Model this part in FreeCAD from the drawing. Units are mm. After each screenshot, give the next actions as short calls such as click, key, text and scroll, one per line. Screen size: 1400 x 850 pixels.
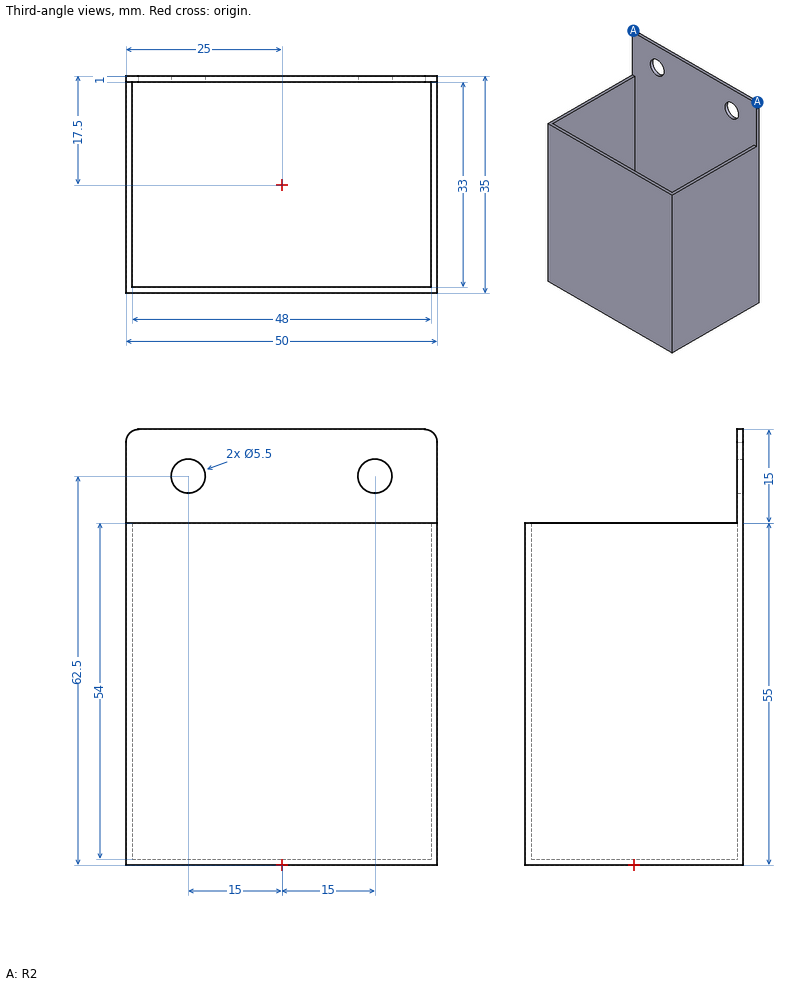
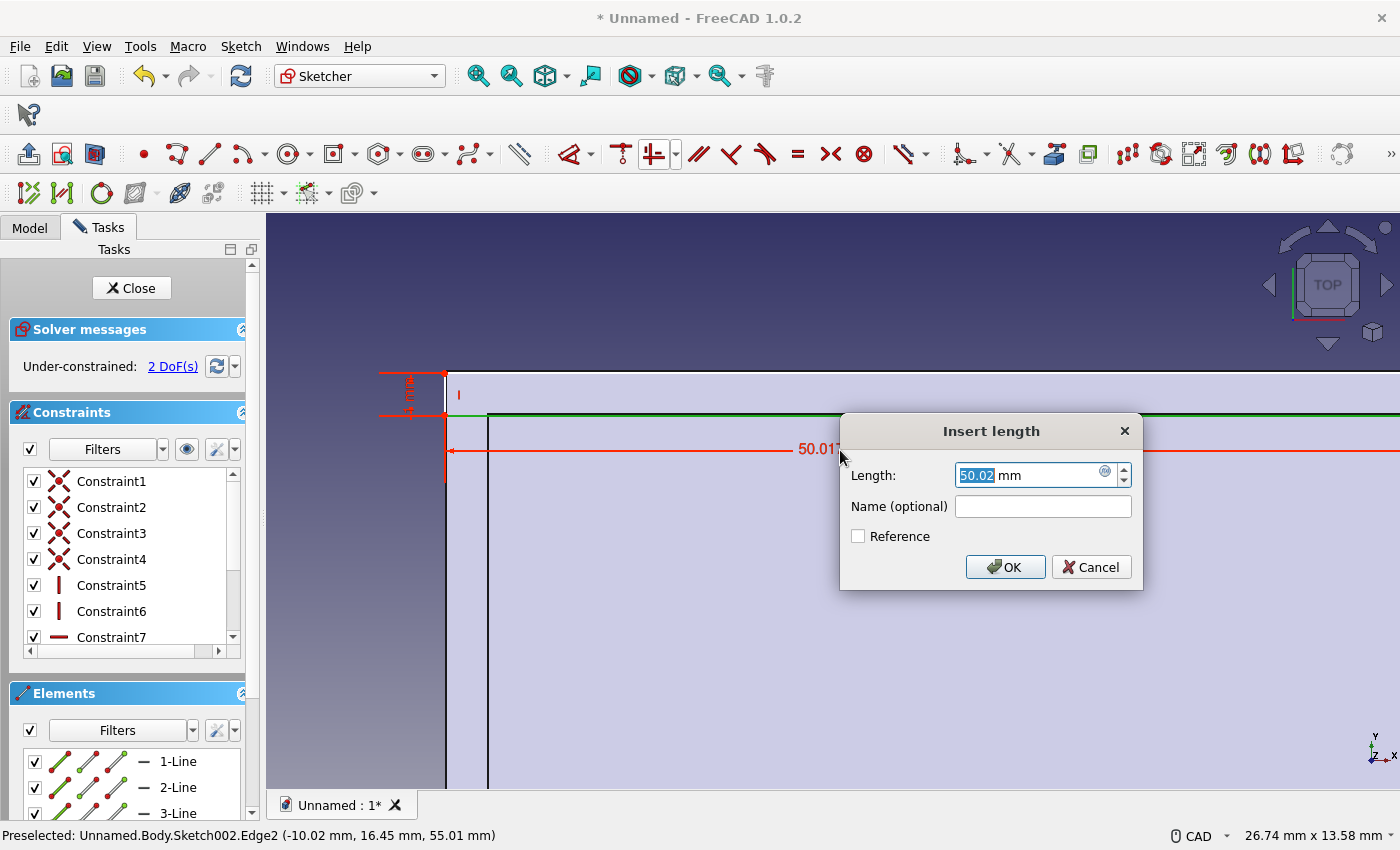
text(50)
key(Return)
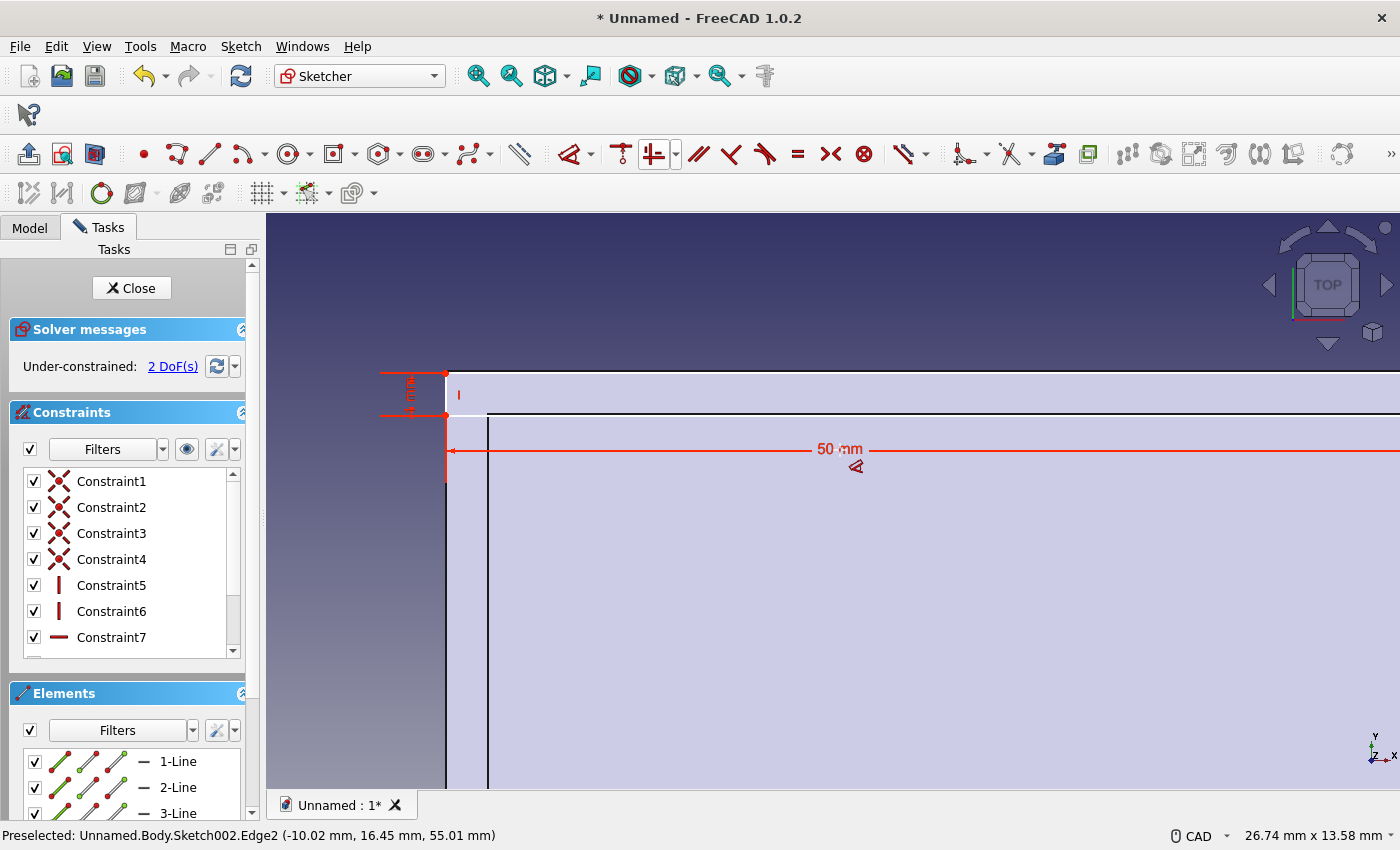
click(446, 373)
click(840, 339)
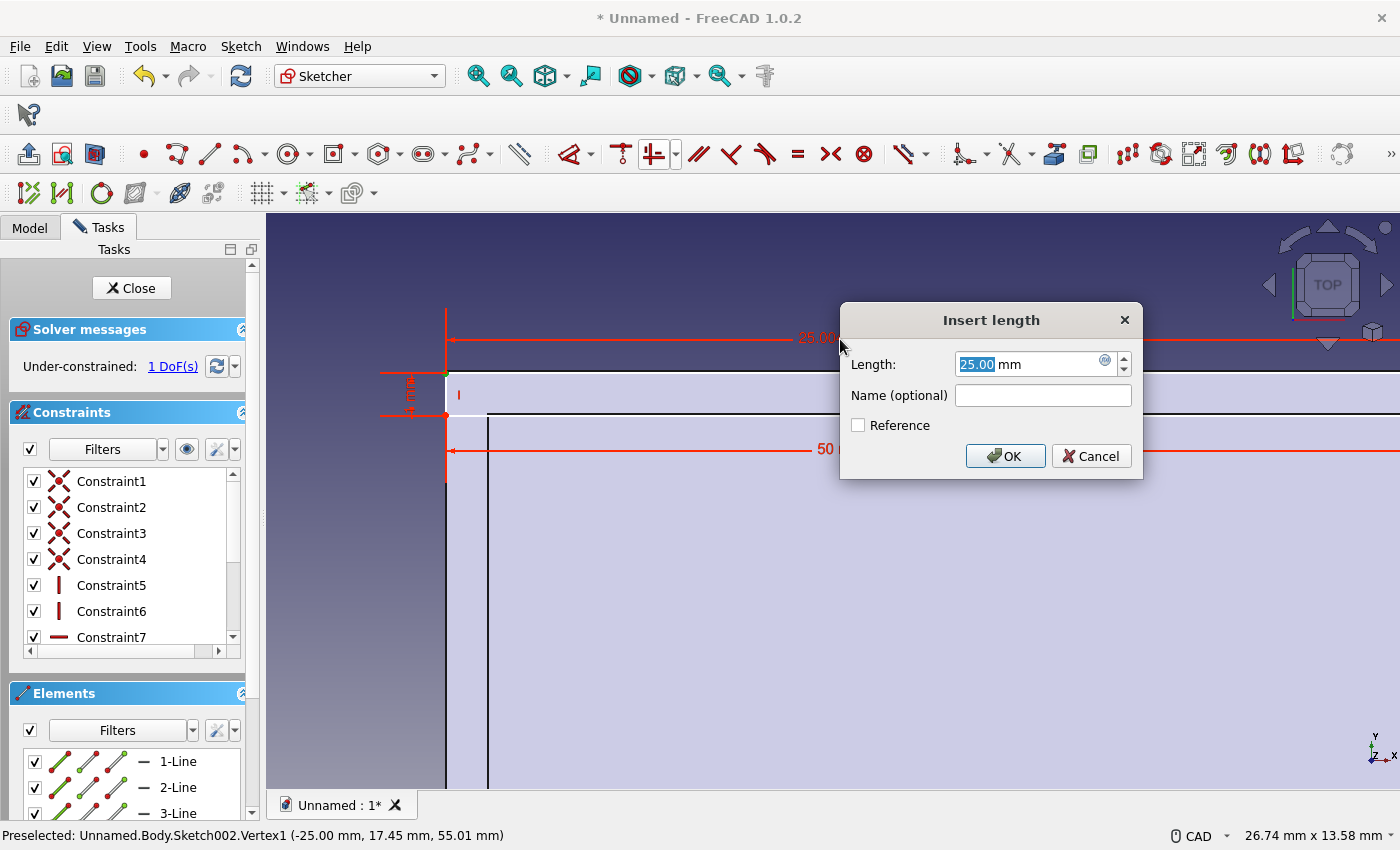
text(25)
key(Return)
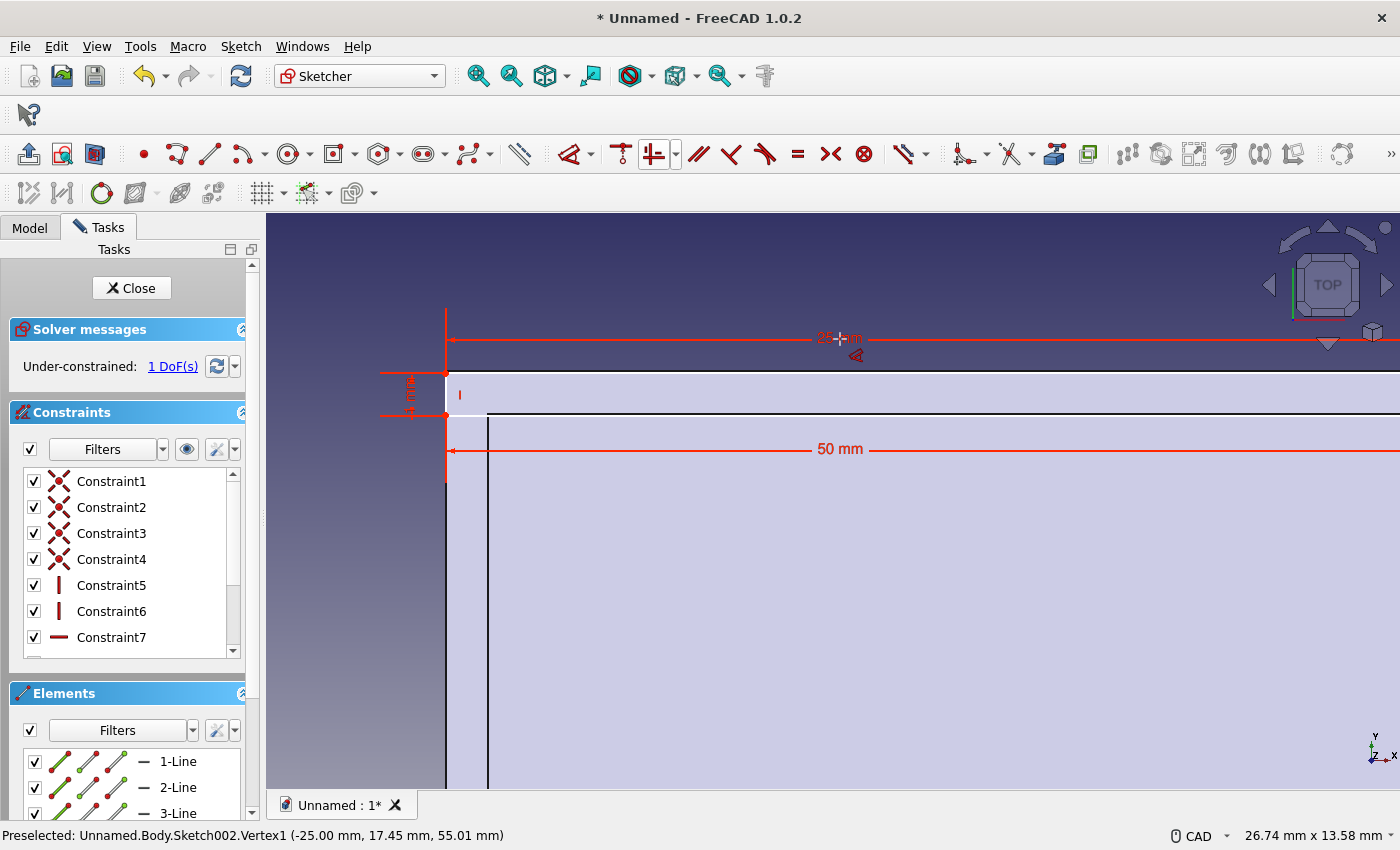
click(446, 373)
click(412, 567)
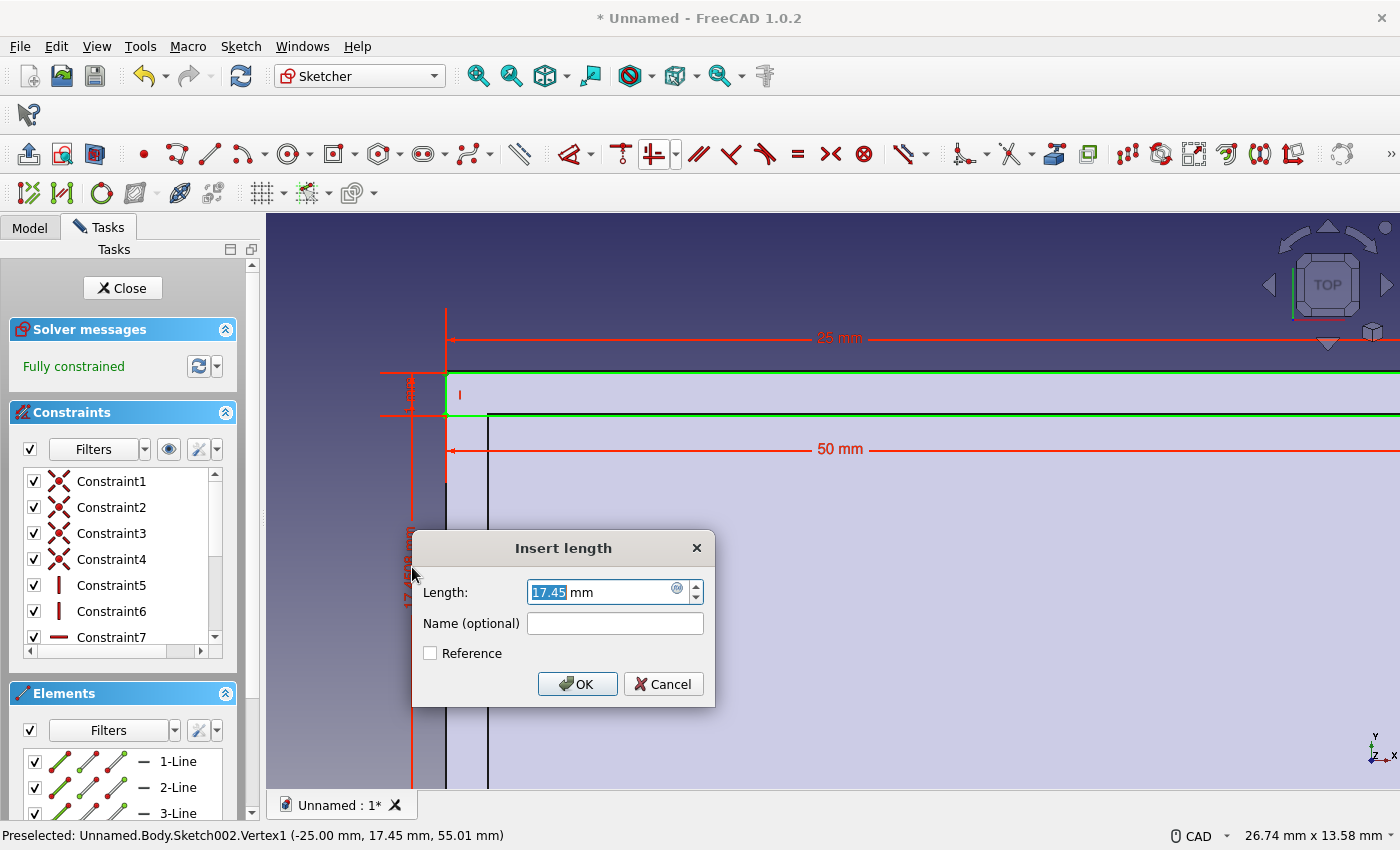
text(17.5)
key(Return)
key(Escape)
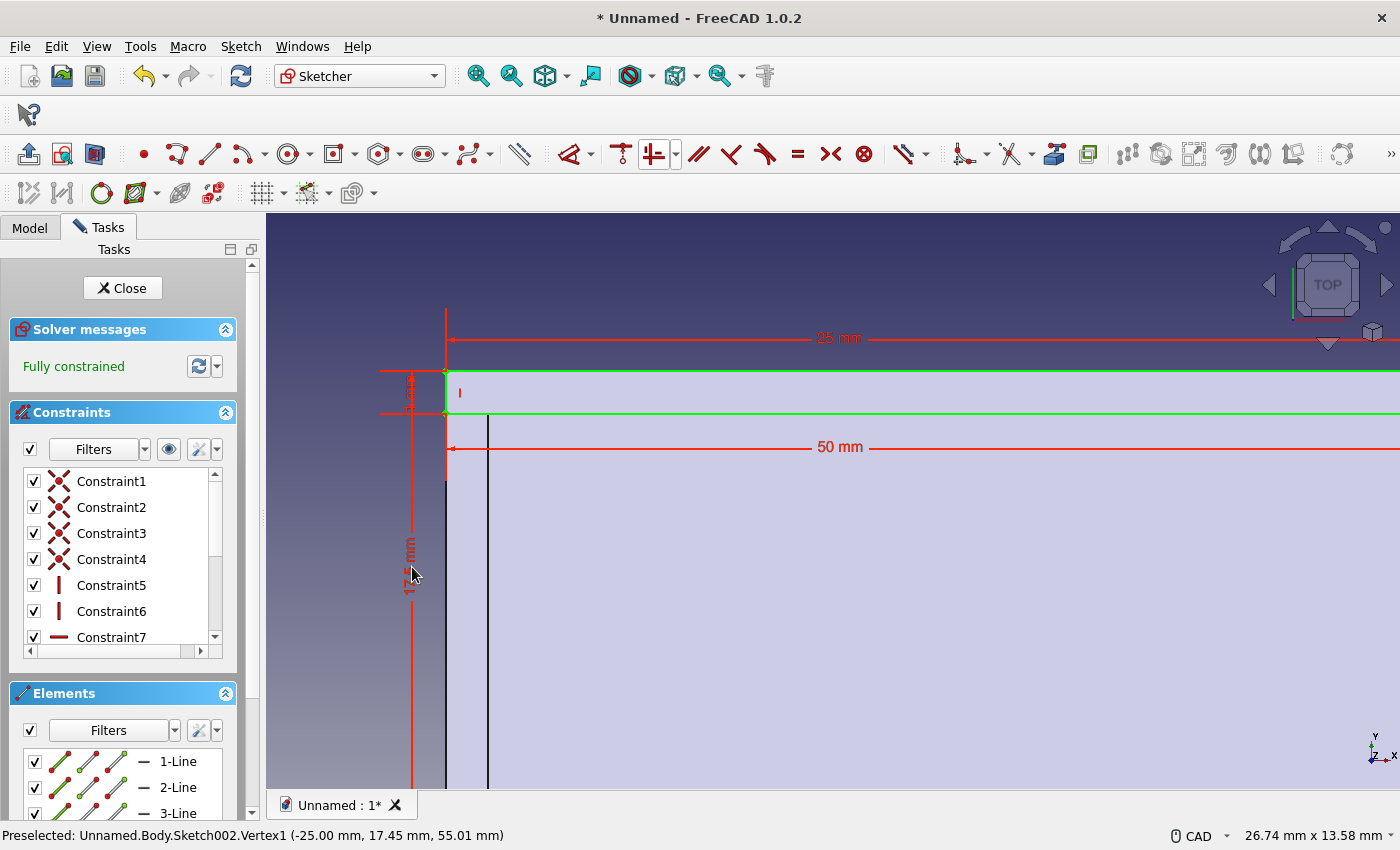
click(123, 288)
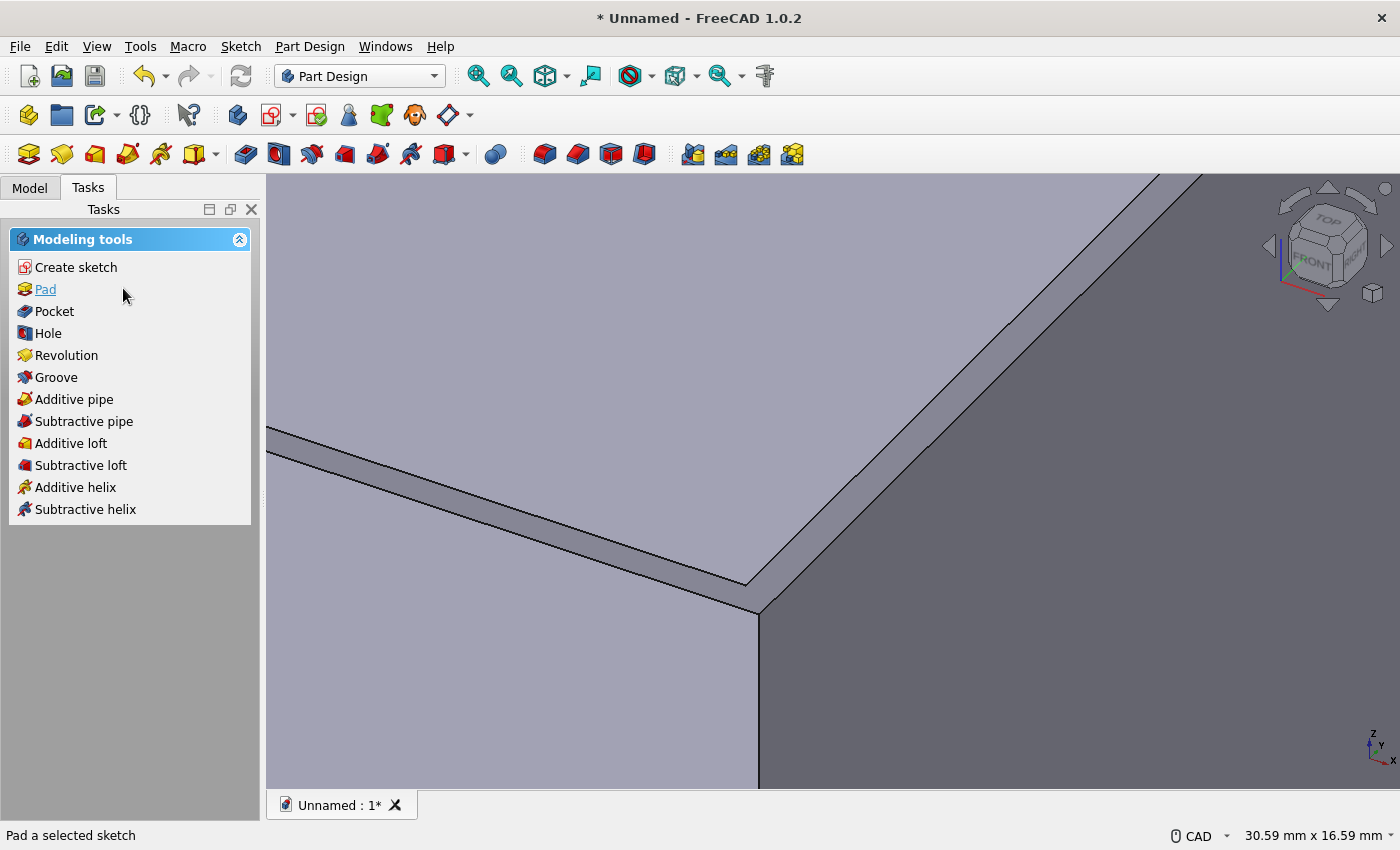
click(29, 154)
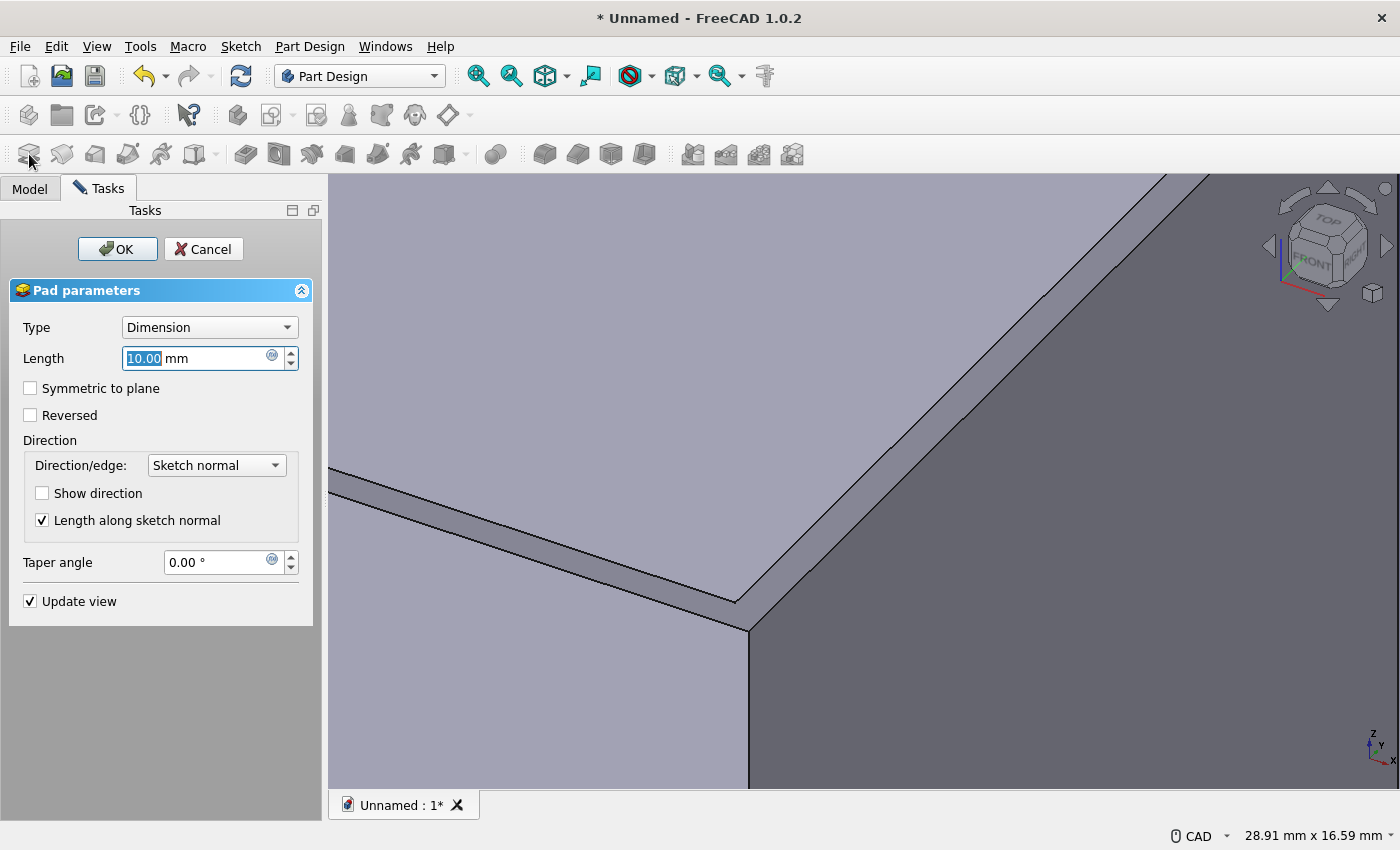
text(15)
key(Tab)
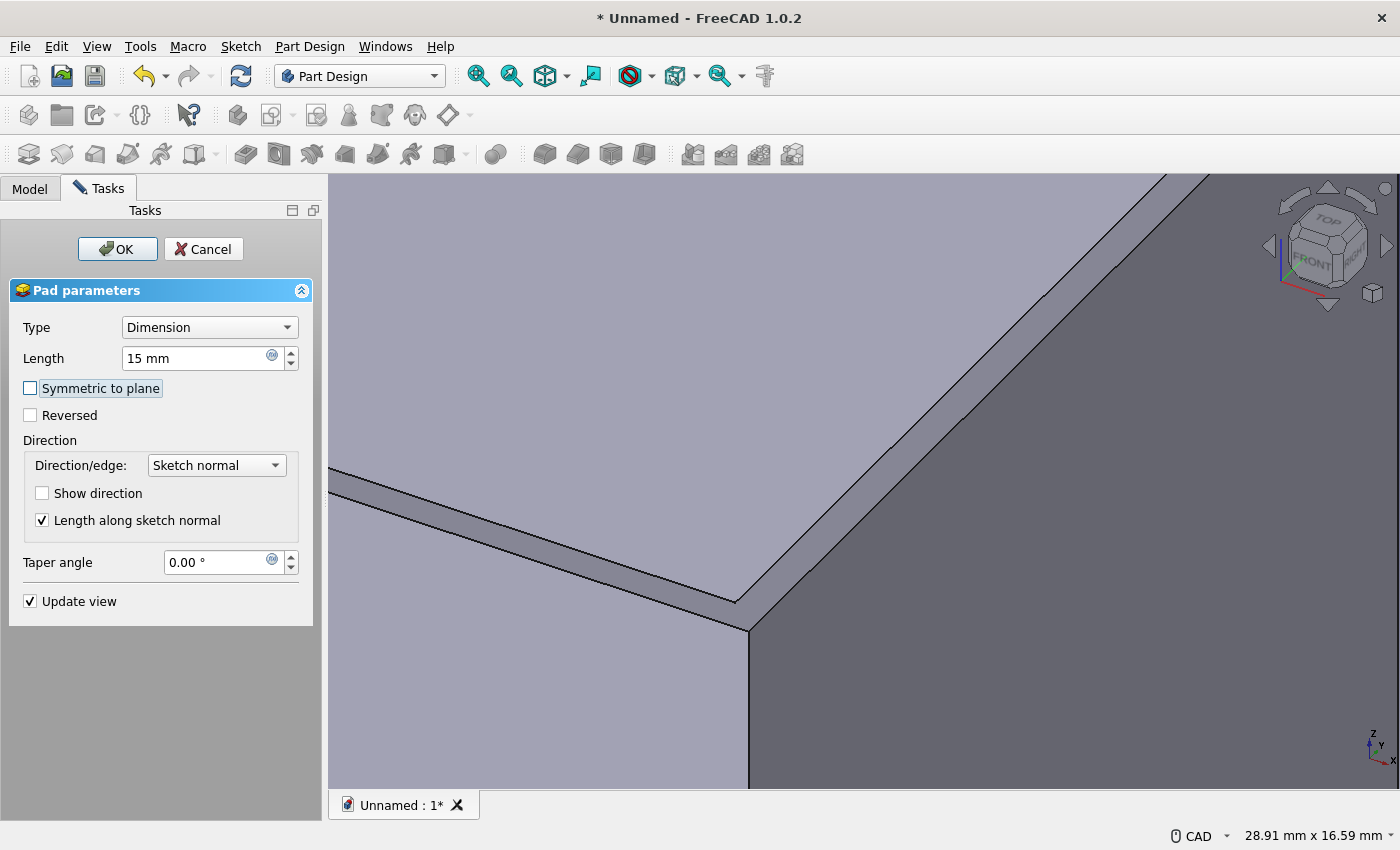
click(118, 249)